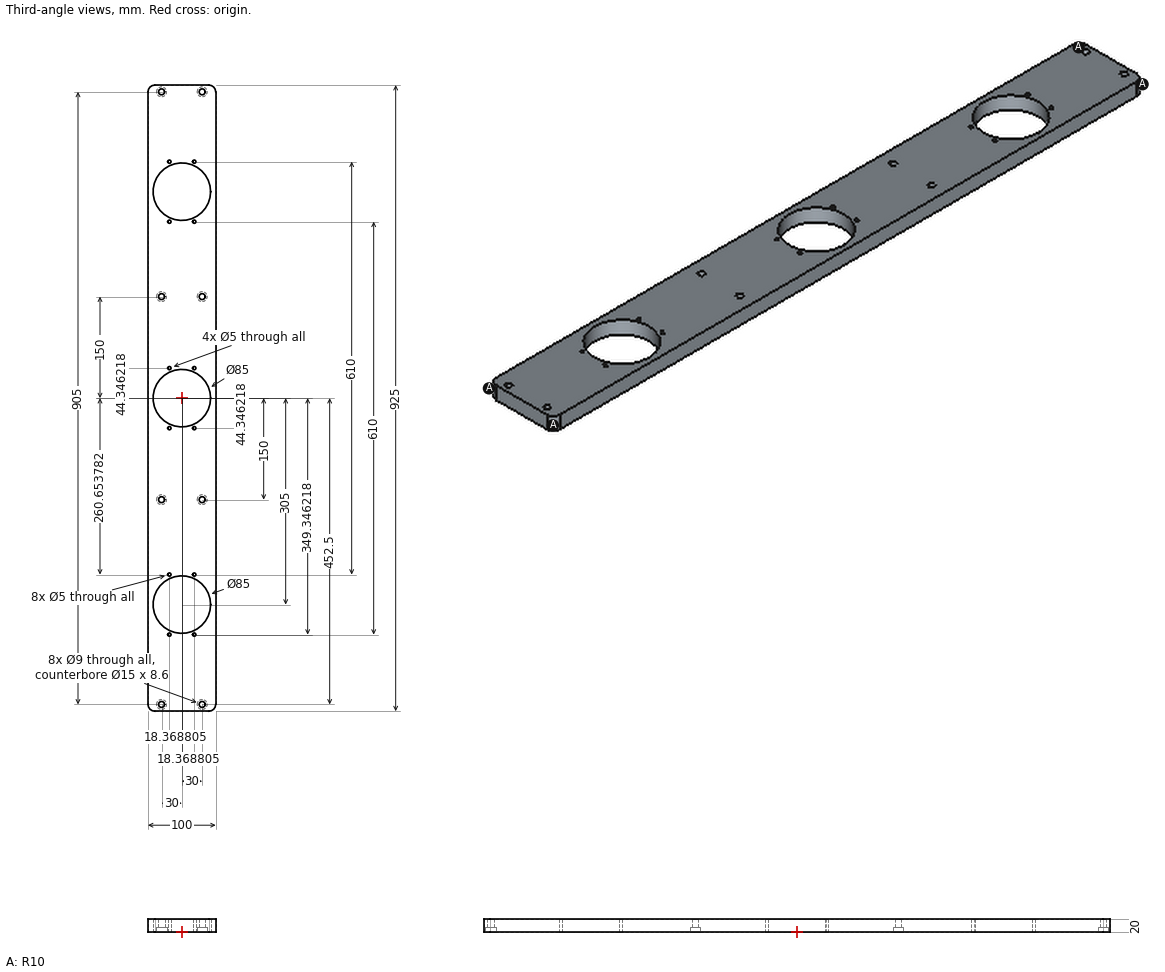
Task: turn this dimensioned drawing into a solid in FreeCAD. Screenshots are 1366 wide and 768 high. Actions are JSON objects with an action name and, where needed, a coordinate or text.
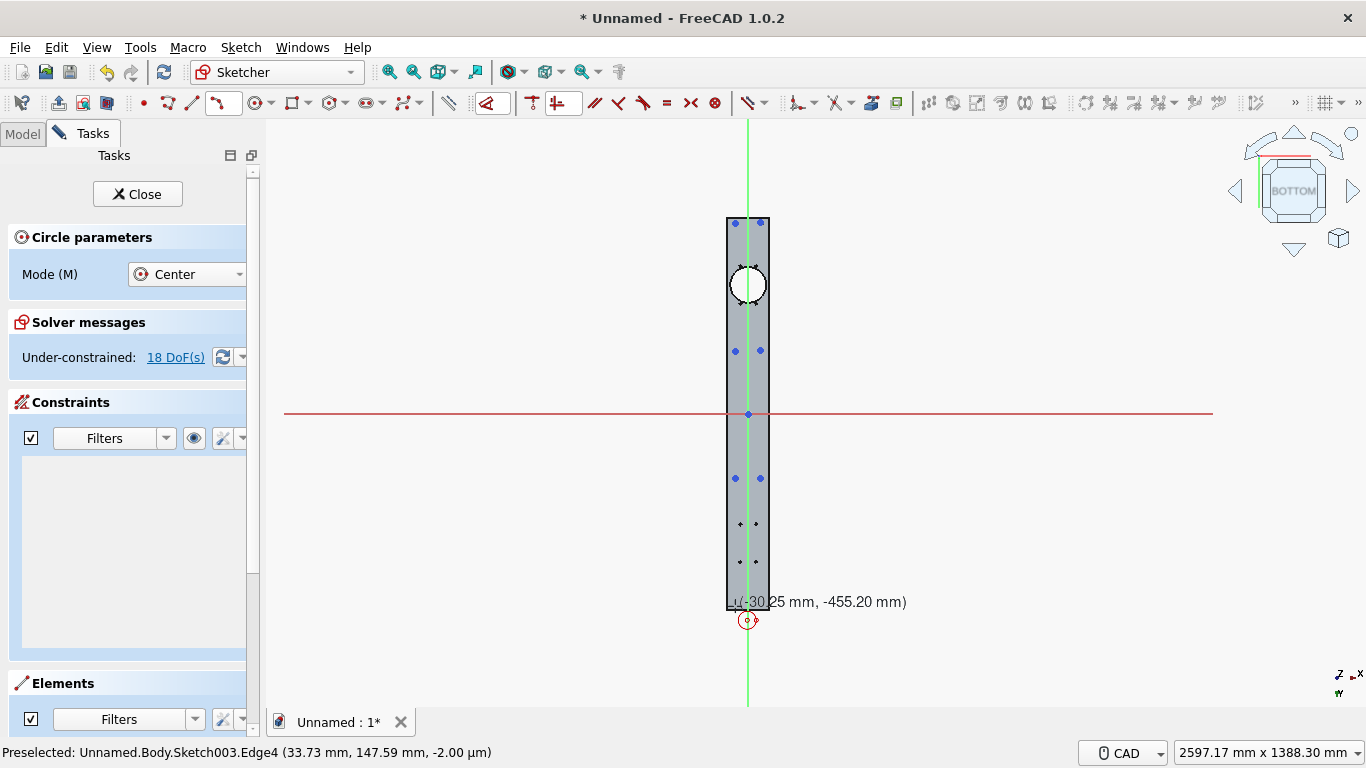
{"action": "scroll", "coordinate": [735, 606], "scroll_direction": "up", "scroll_amount": 2}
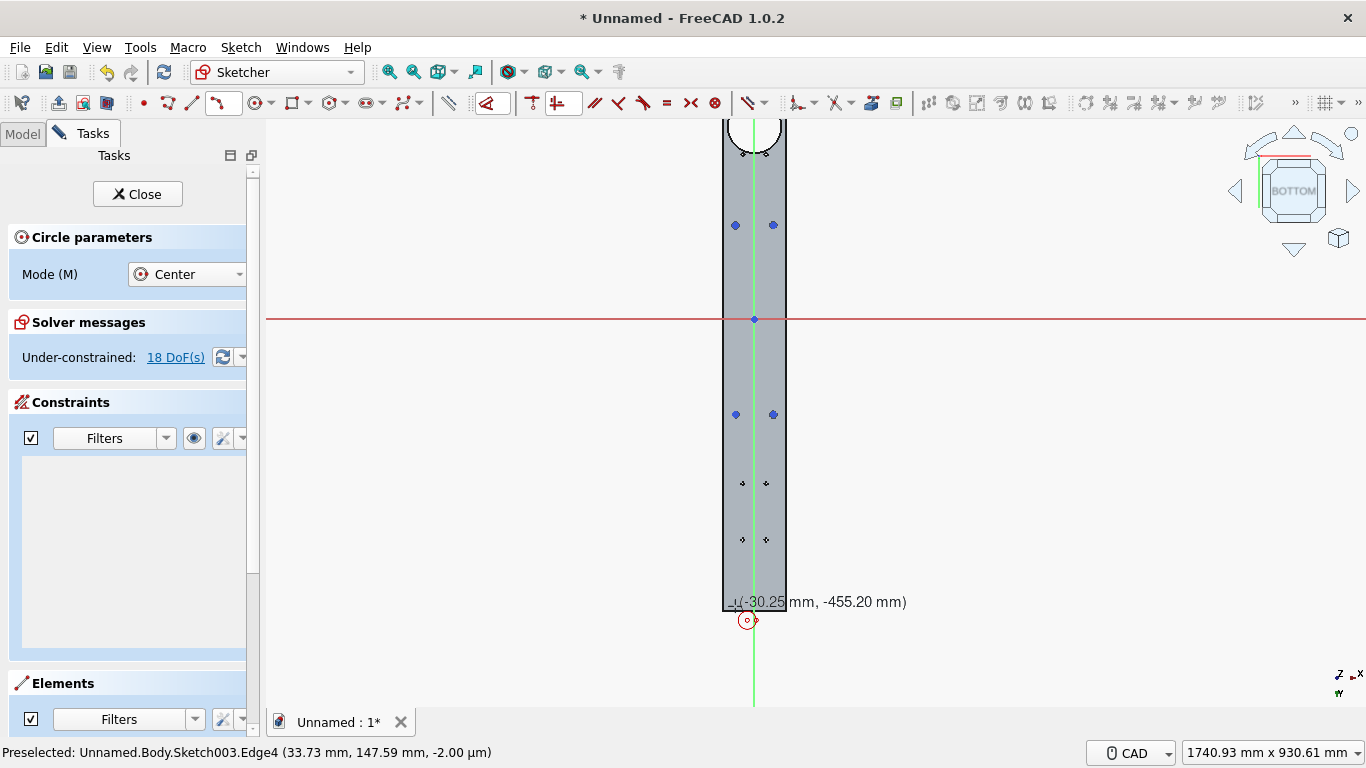
{"action": "left_click", "coordinate": [736, 605]}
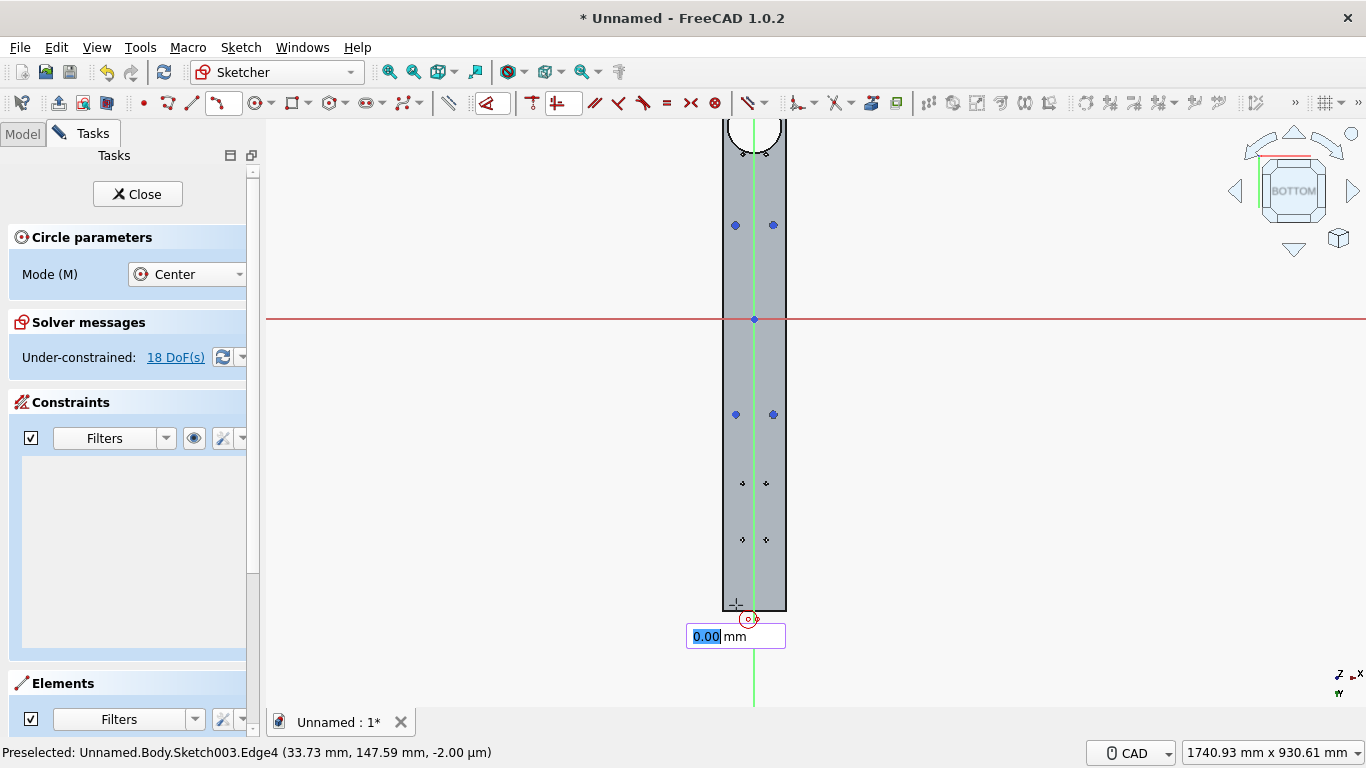
{"action": "scroll", "coordinate": [738, 603], "scroll_direction": "up", "scroll_amount": 9}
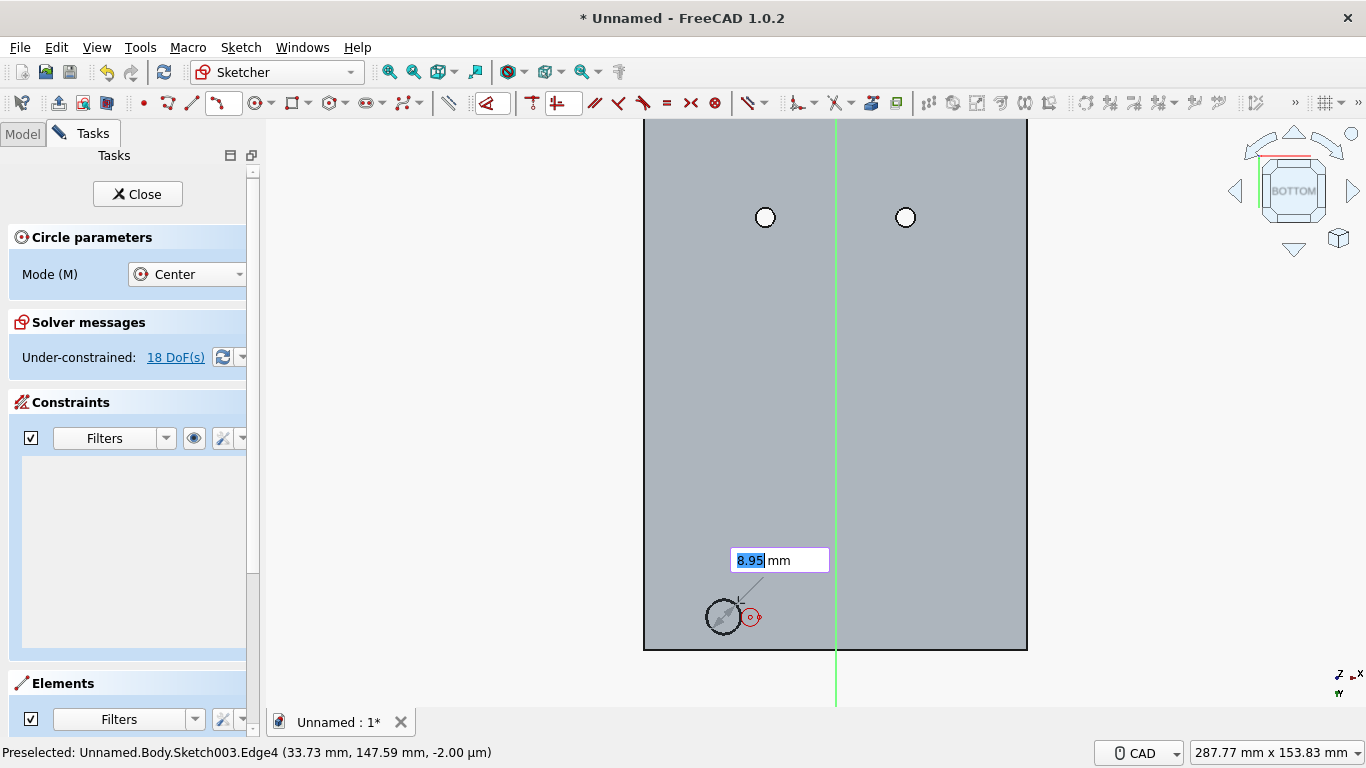
{"action": "left_click", "coordinate": [733, 600]}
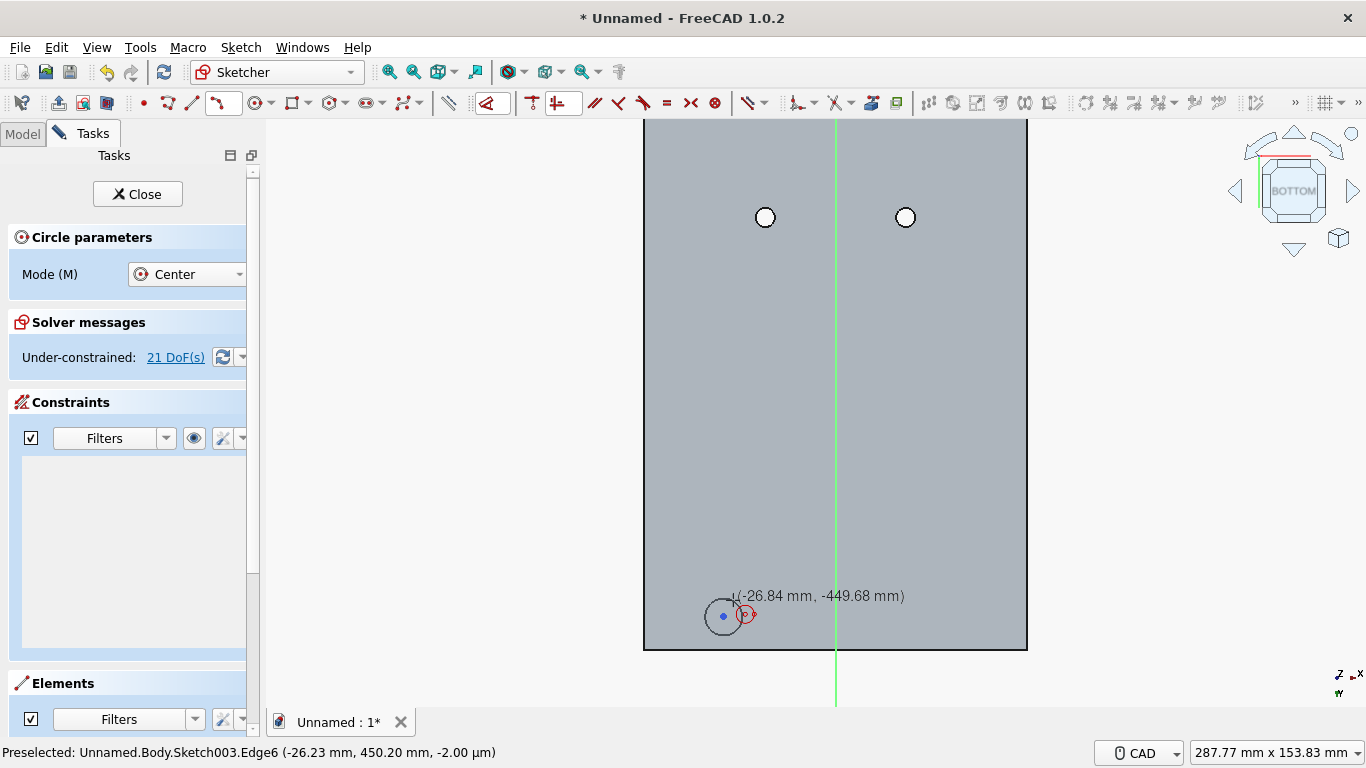
{"action": "scroll", "coordinate": [950, 612], "scroll_direction": "up", "scroll_amount": 2}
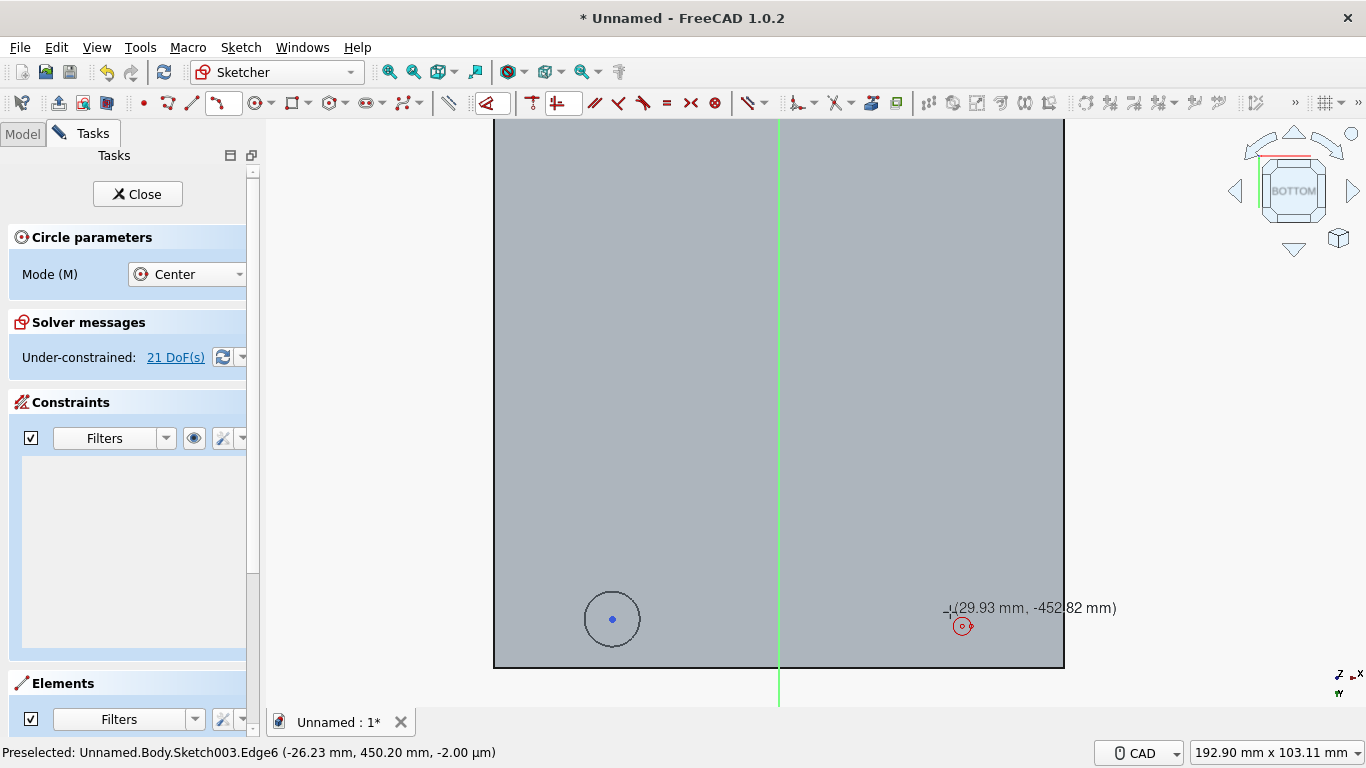
{"action": "scroll", "coordinate": [745, 604], "scroll_direction": "down", "scroll_amount": 13}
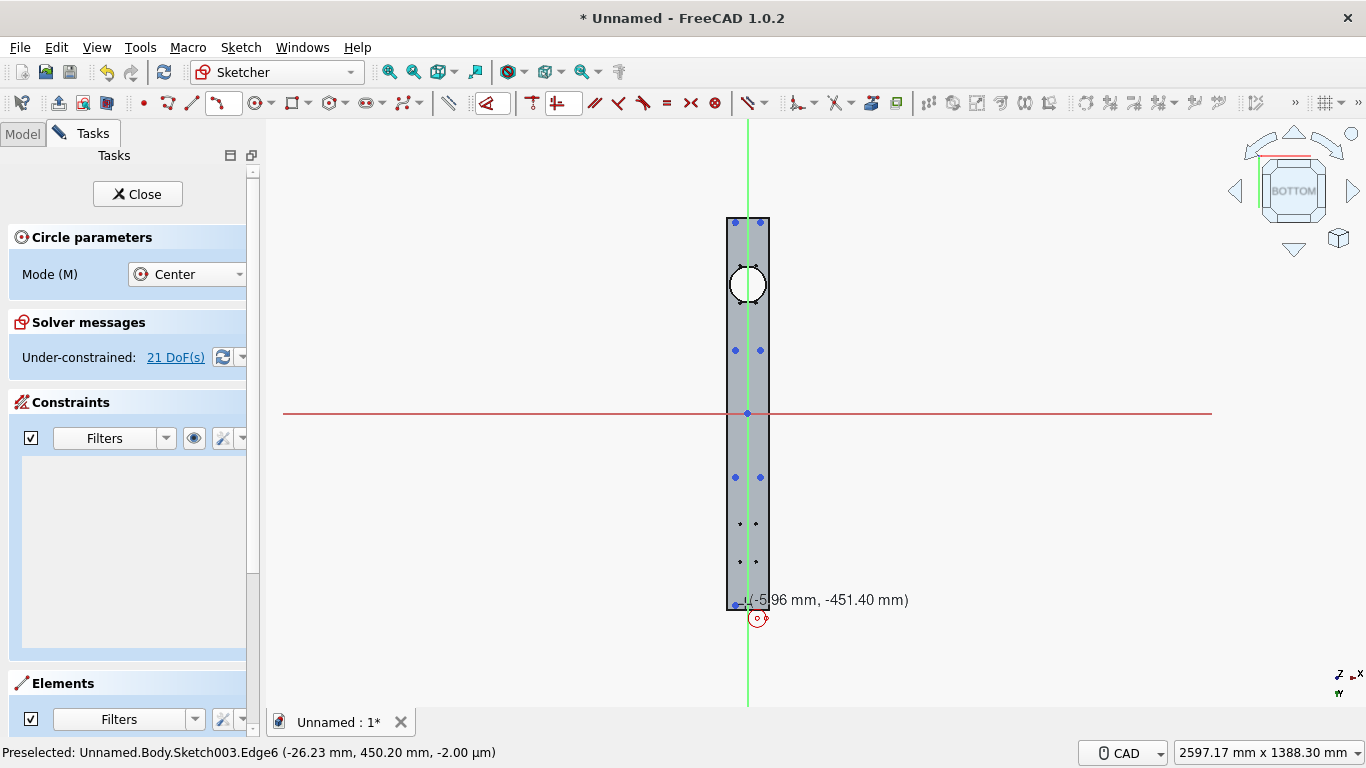
{"action": "scroll", "coordinate": [761, 605], "scroll_direction": "up", "scroll_amount": 2}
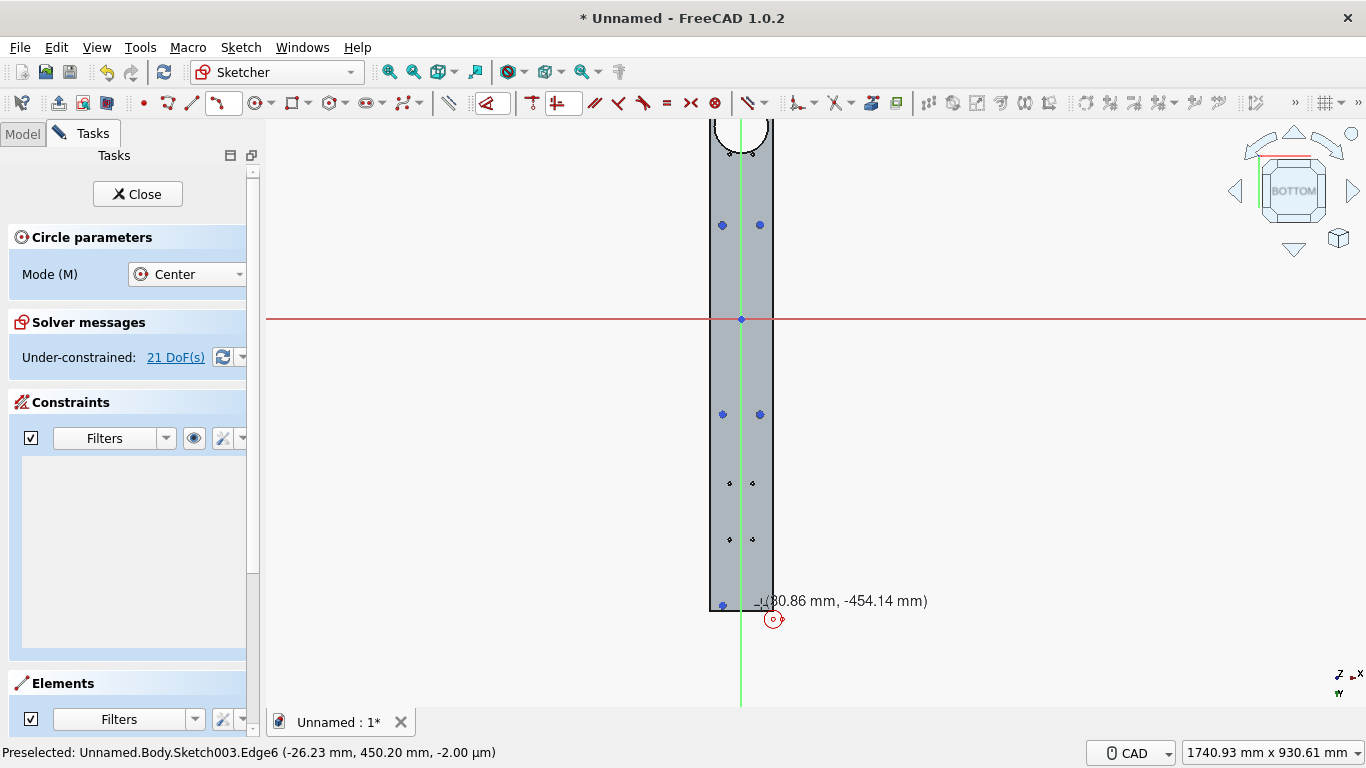
{"action": "left_click", "coordinate": [760, 605]}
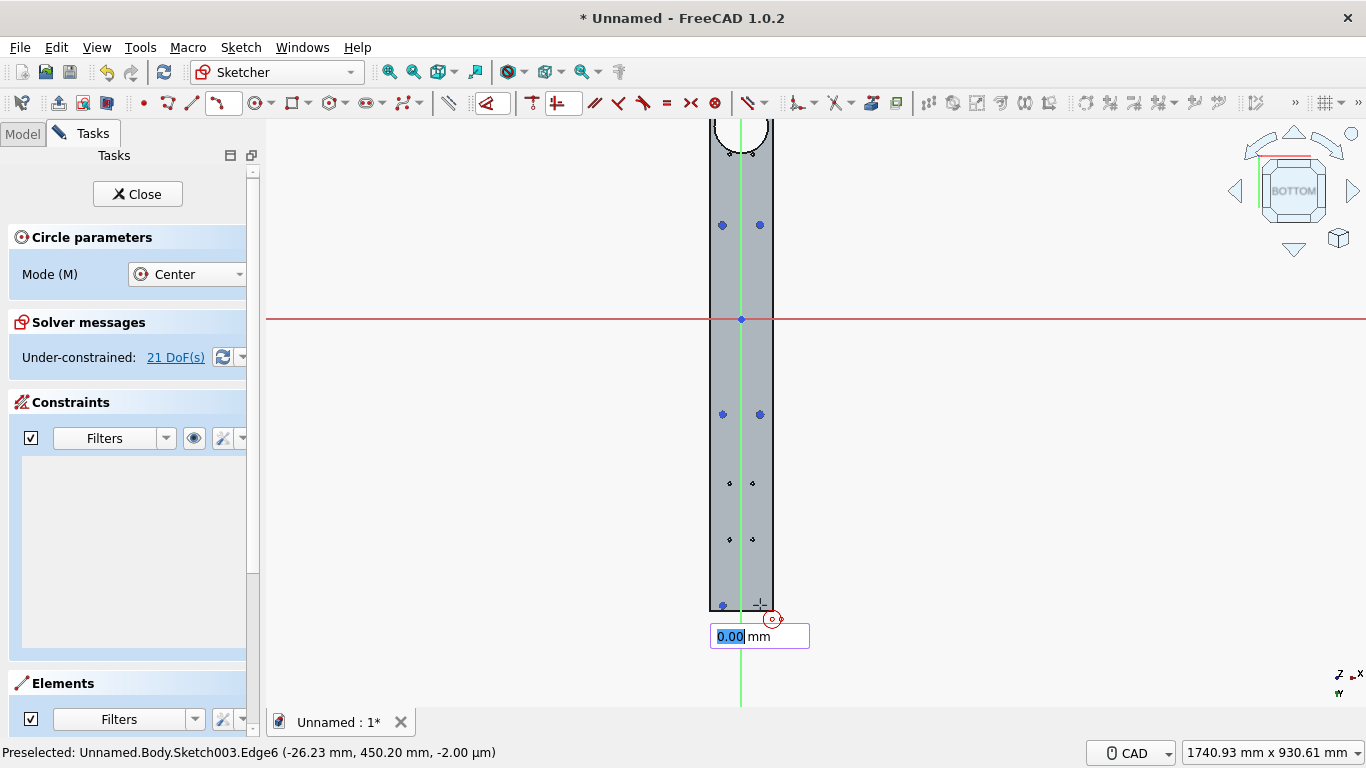
{"action": "scroll", "coordinate": [762, 603], "scroll_direction": "up", "scroll_amount": 9}